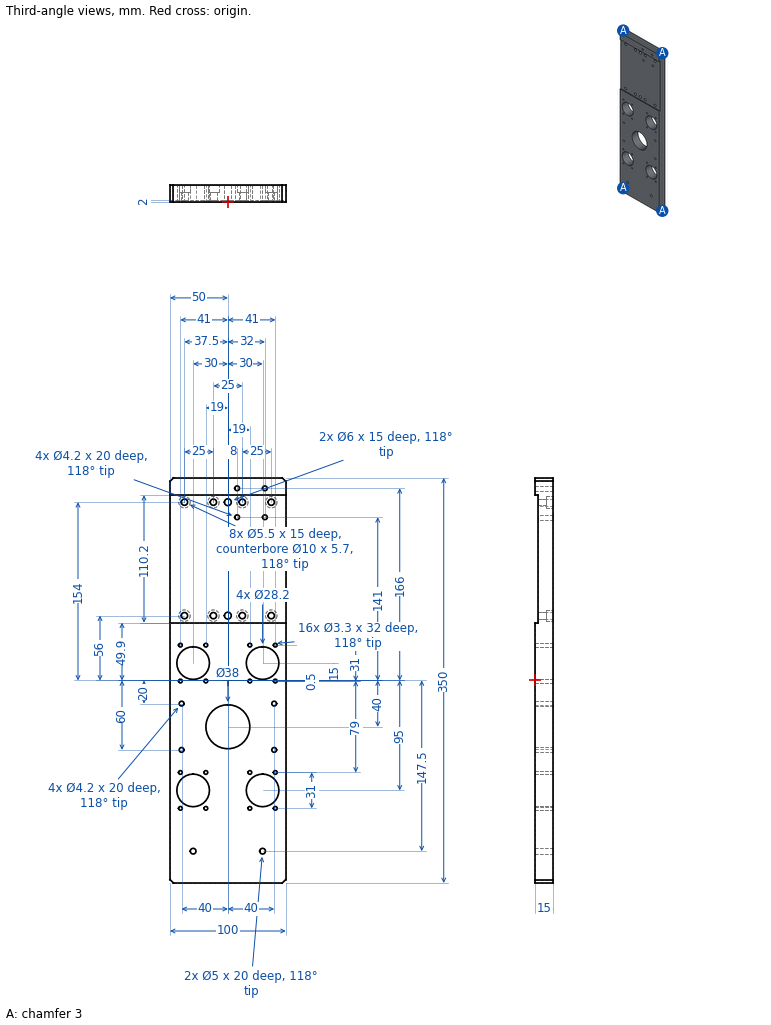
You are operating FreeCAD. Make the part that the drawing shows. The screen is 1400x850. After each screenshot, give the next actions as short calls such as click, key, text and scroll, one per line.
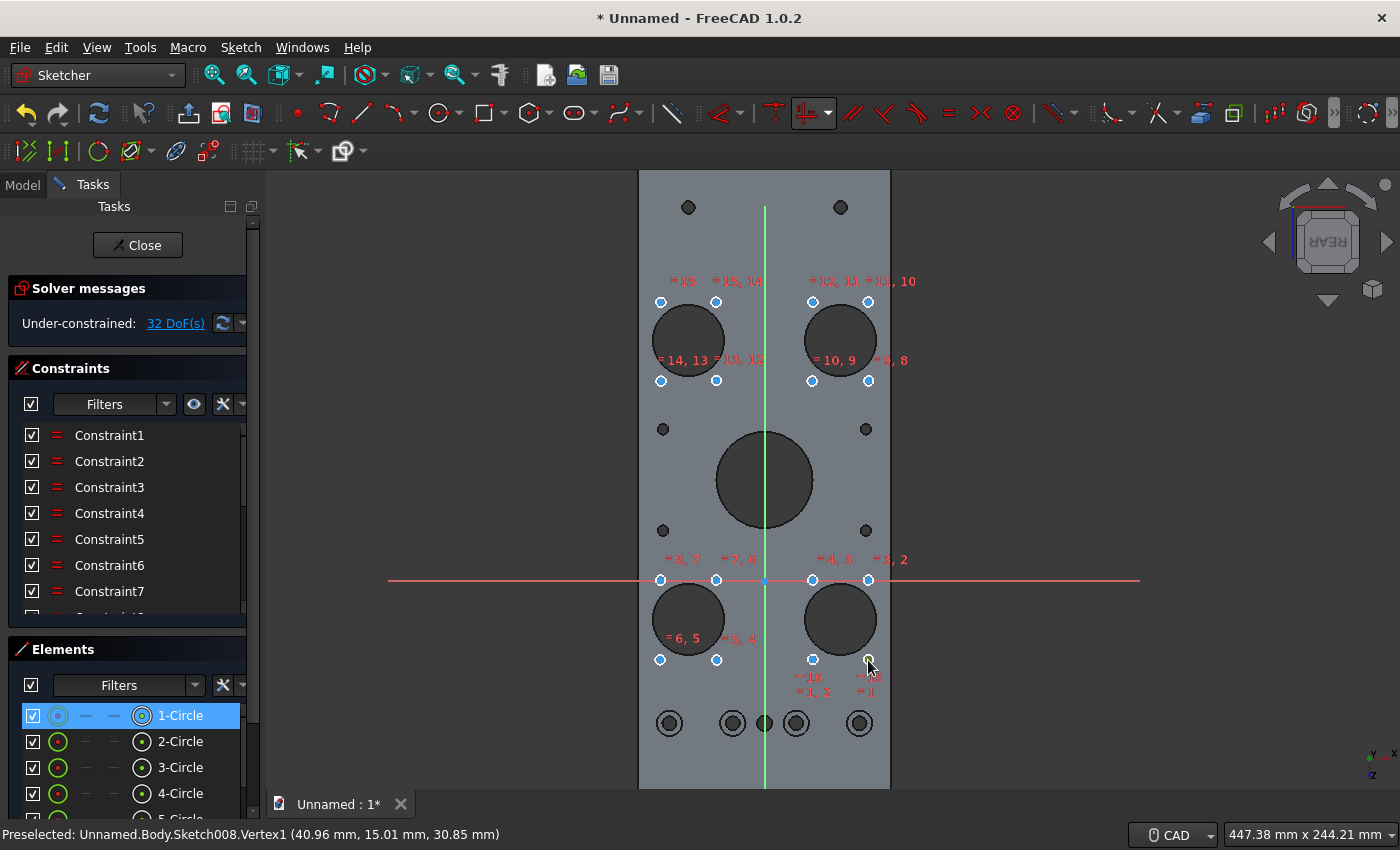
click(868, 580)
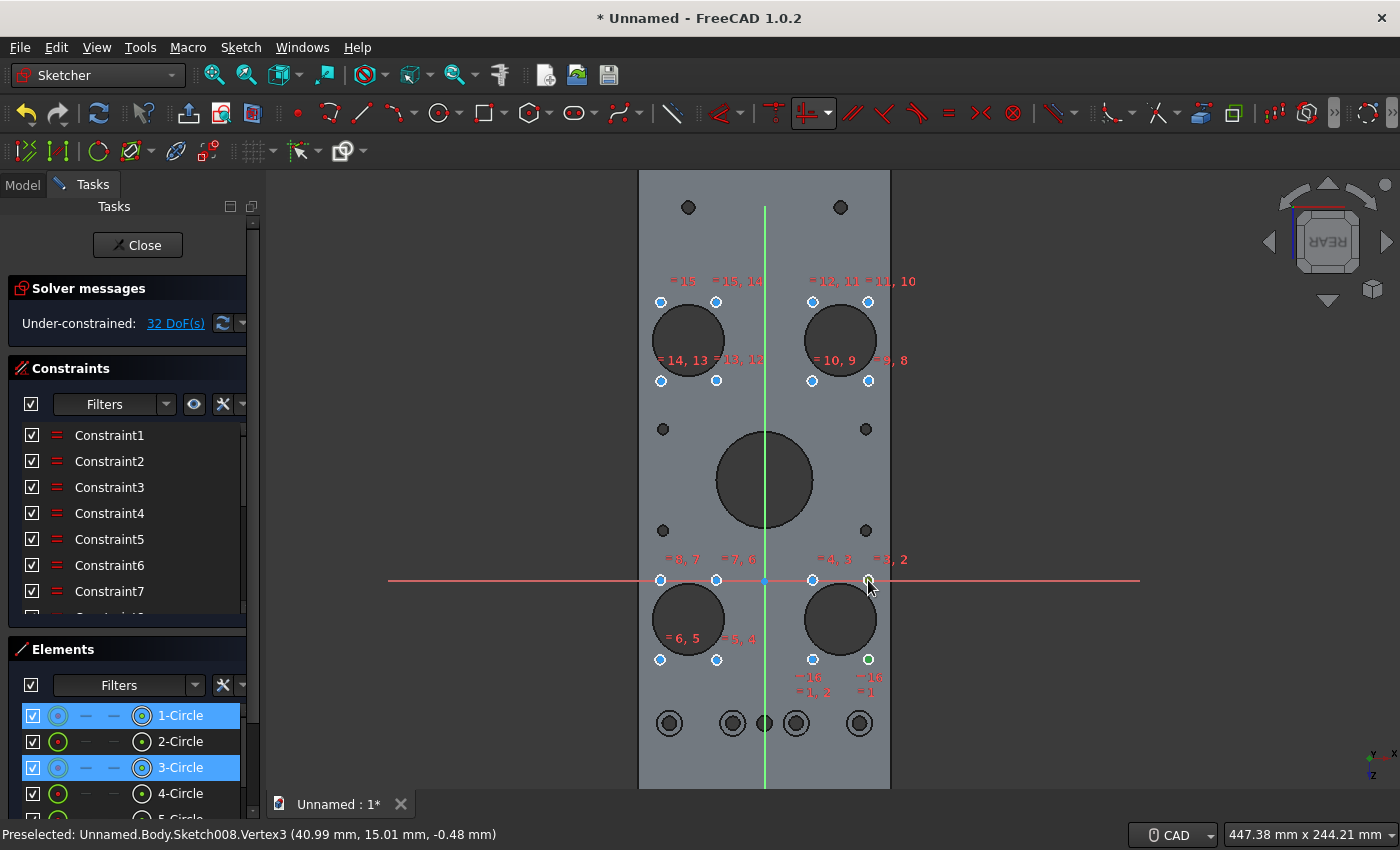
key(v)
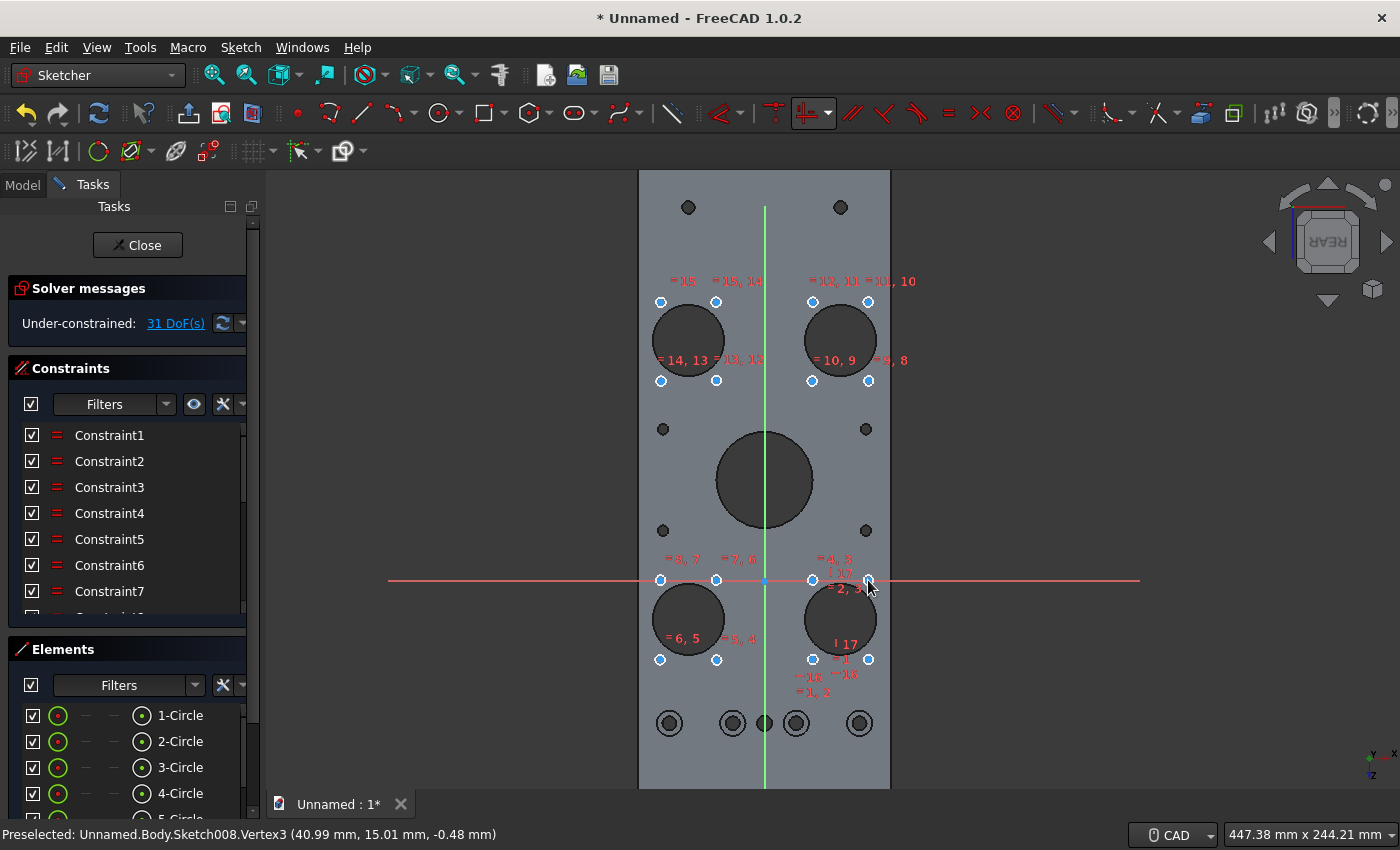
click(813, 660)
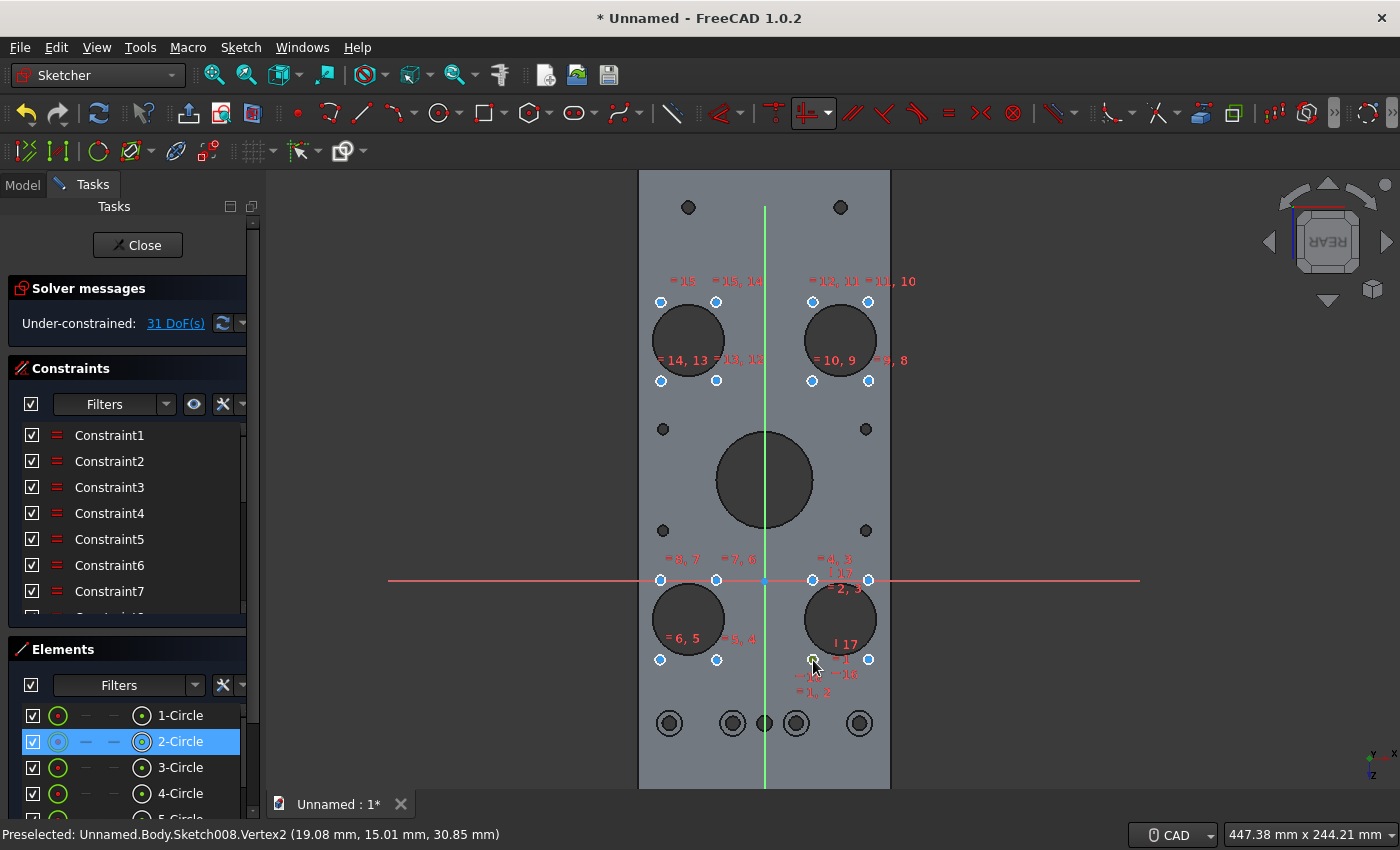
click(813, 580)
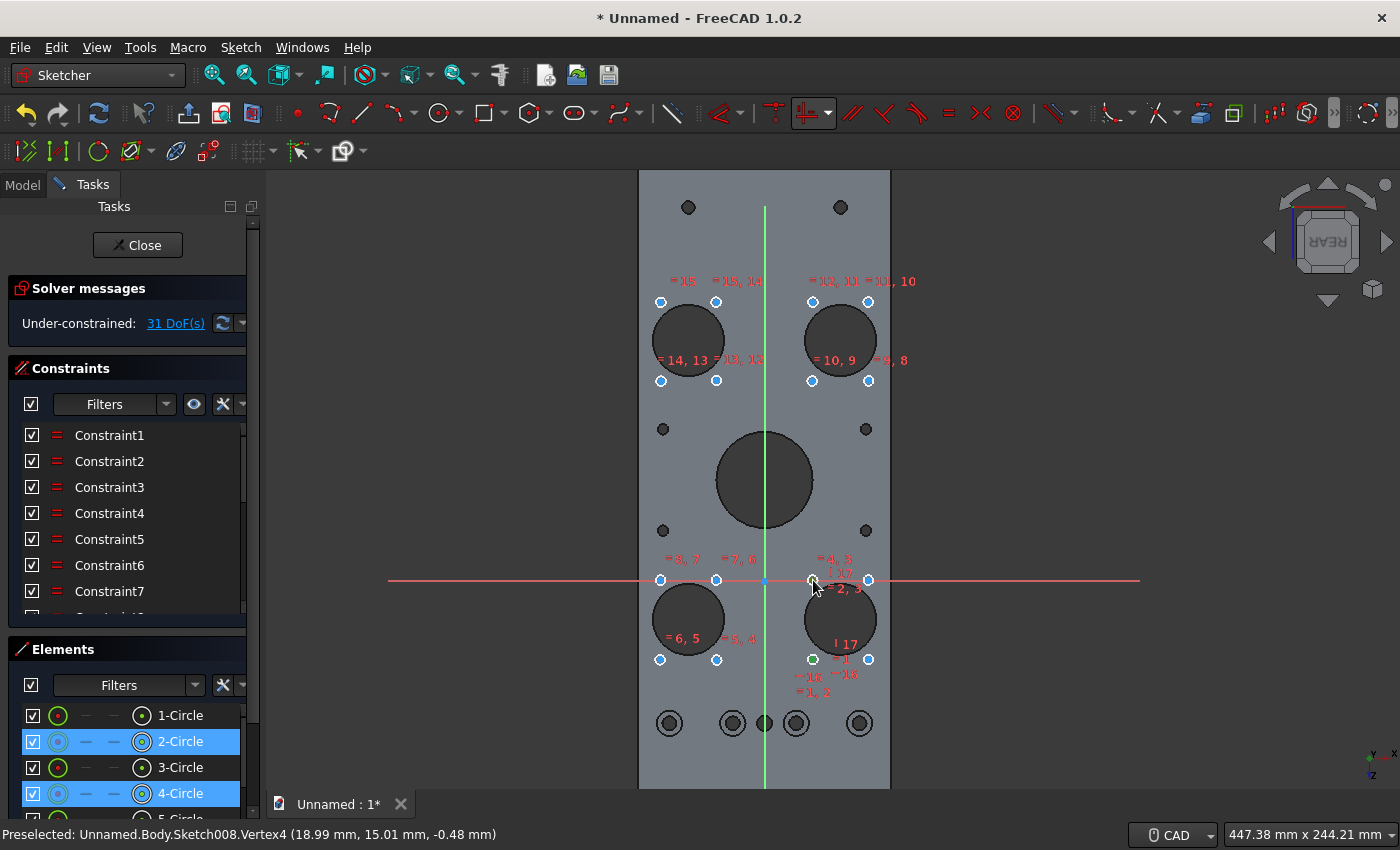
key(v)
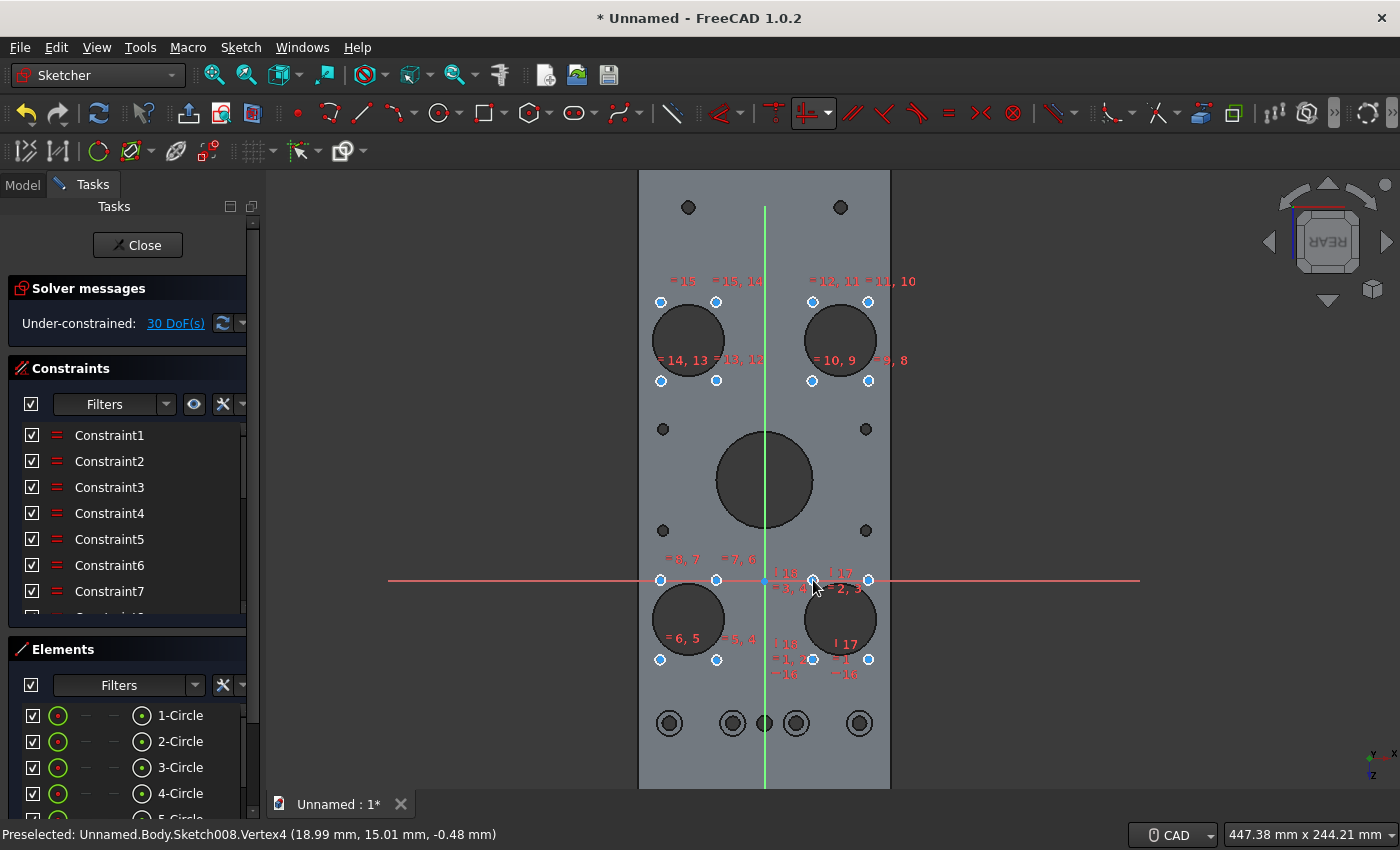
click(868, 580)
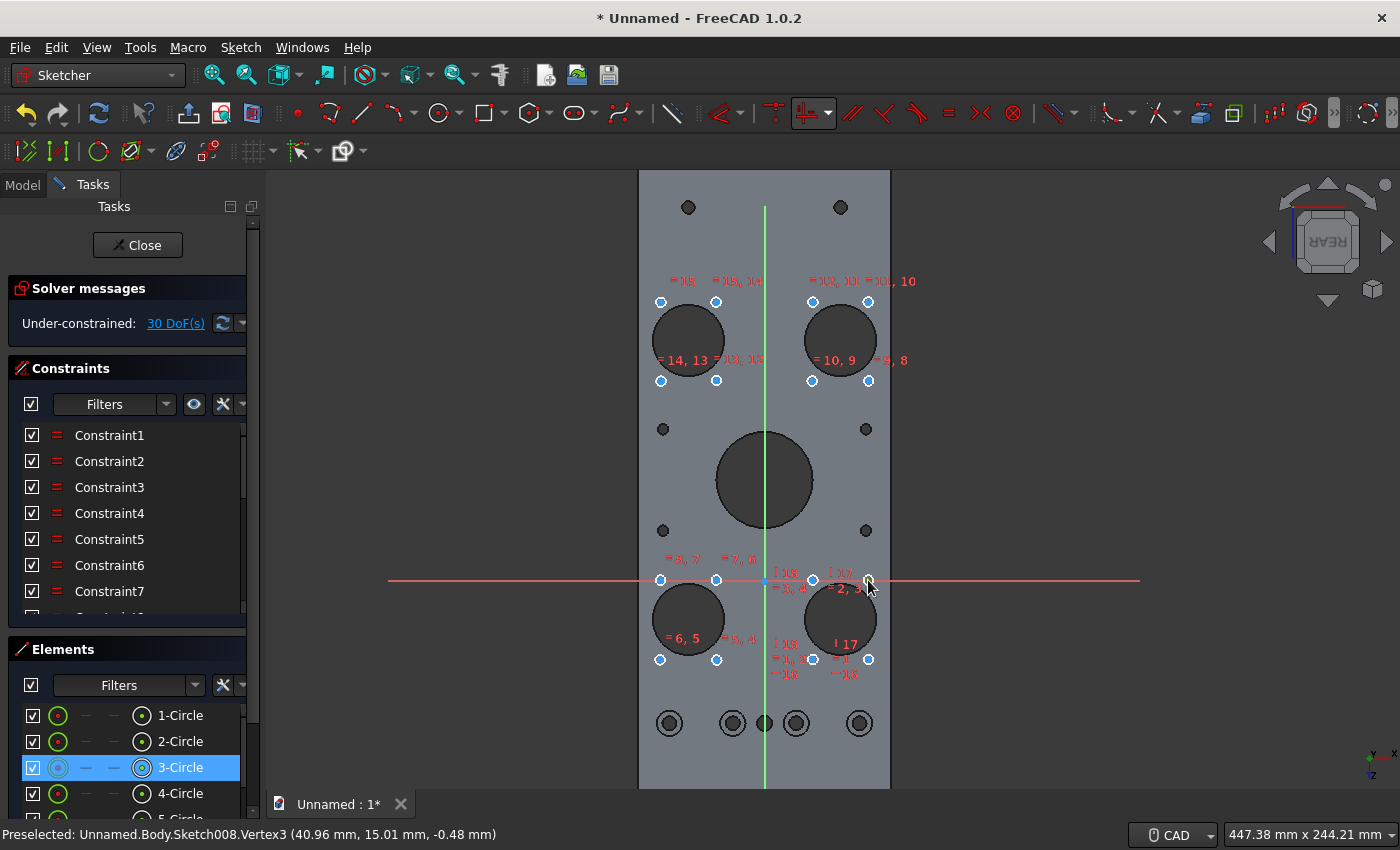
click(813, 580)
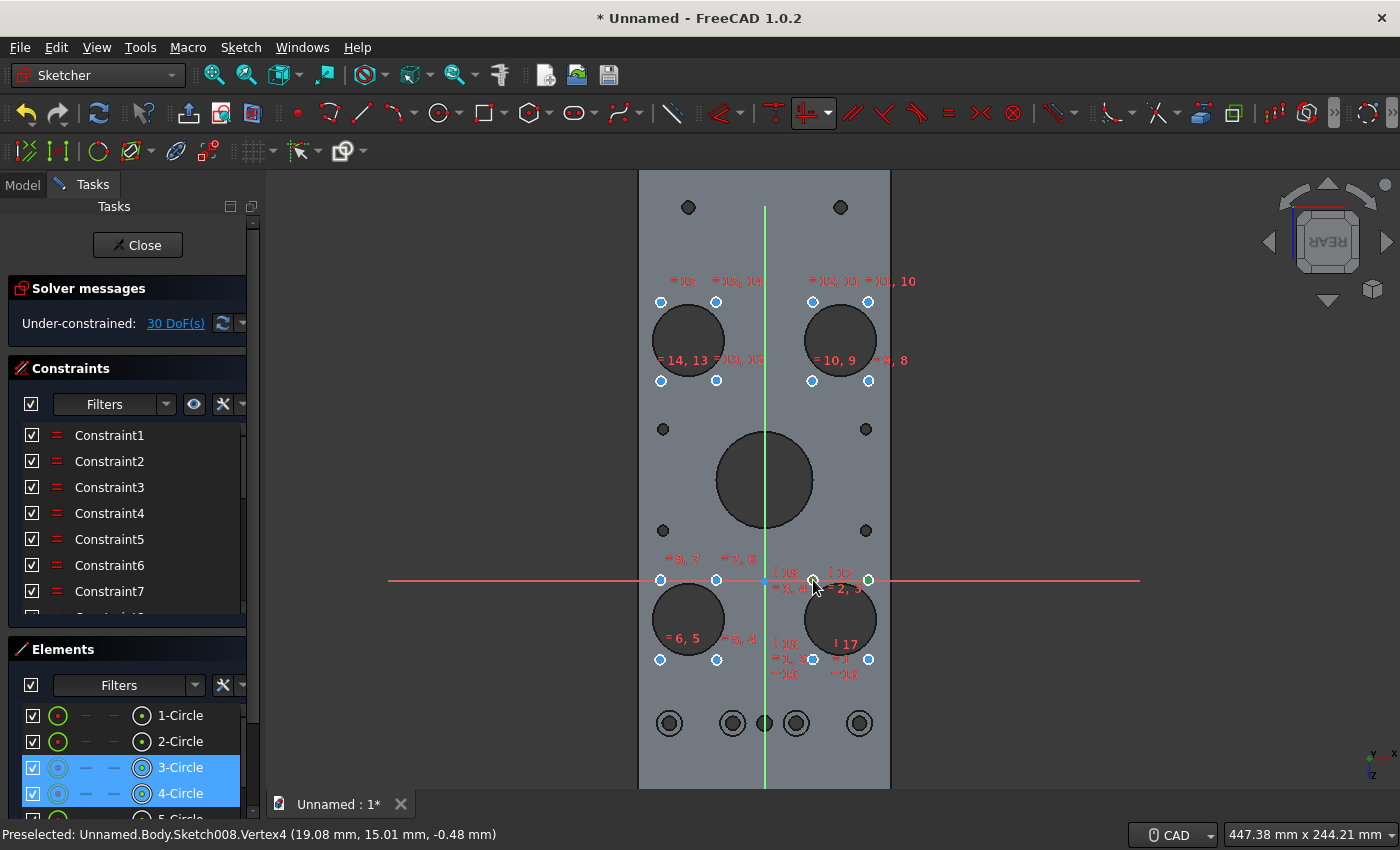
key(h)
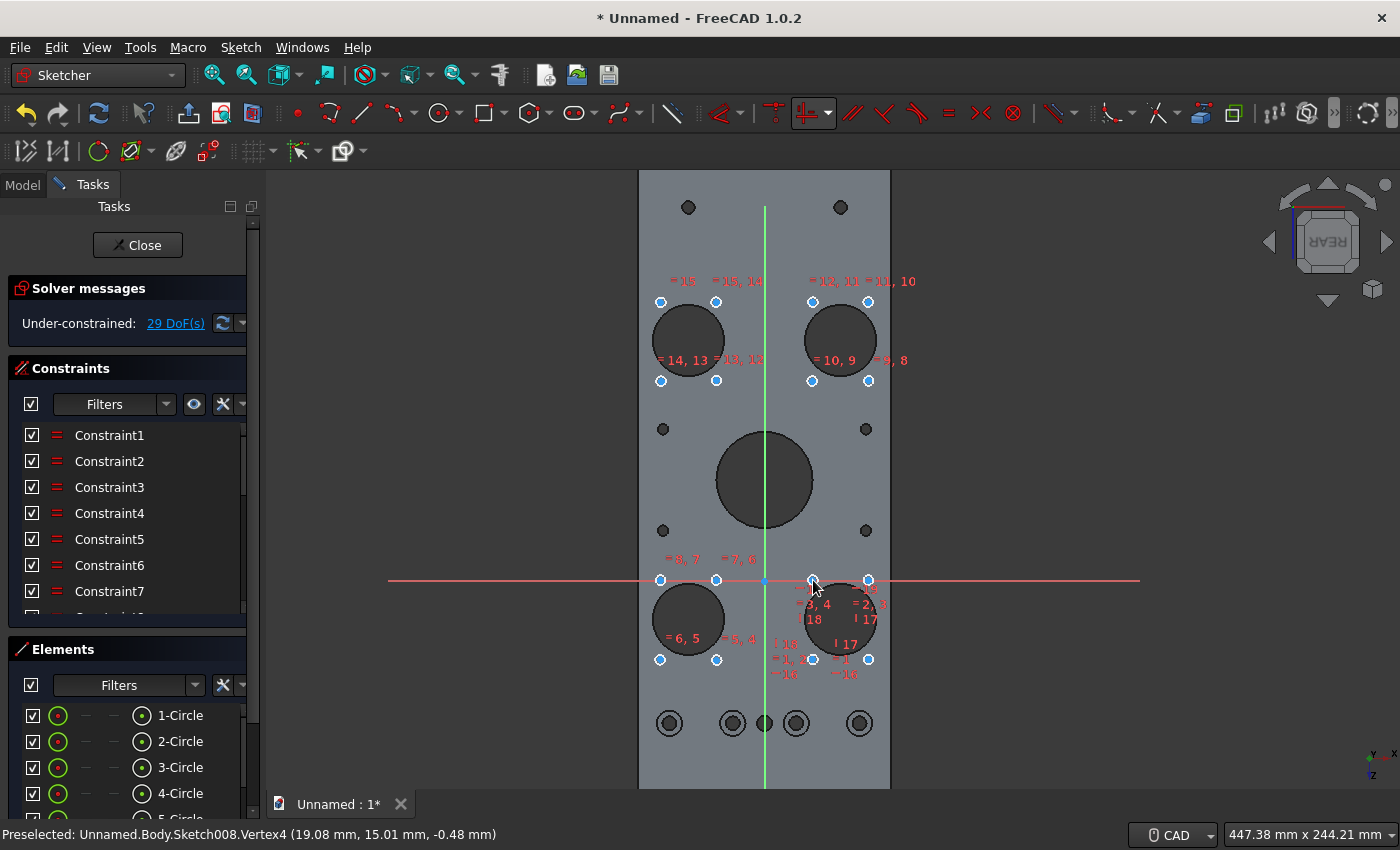
click(813, 660)